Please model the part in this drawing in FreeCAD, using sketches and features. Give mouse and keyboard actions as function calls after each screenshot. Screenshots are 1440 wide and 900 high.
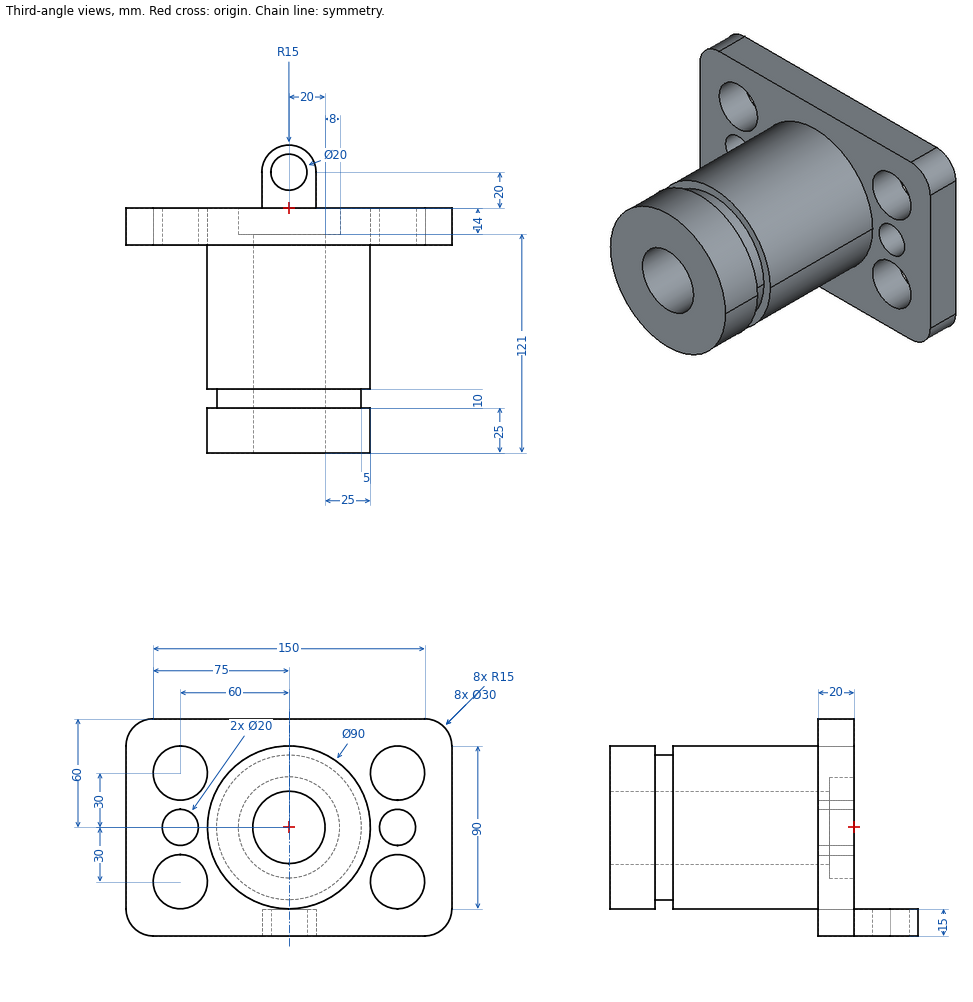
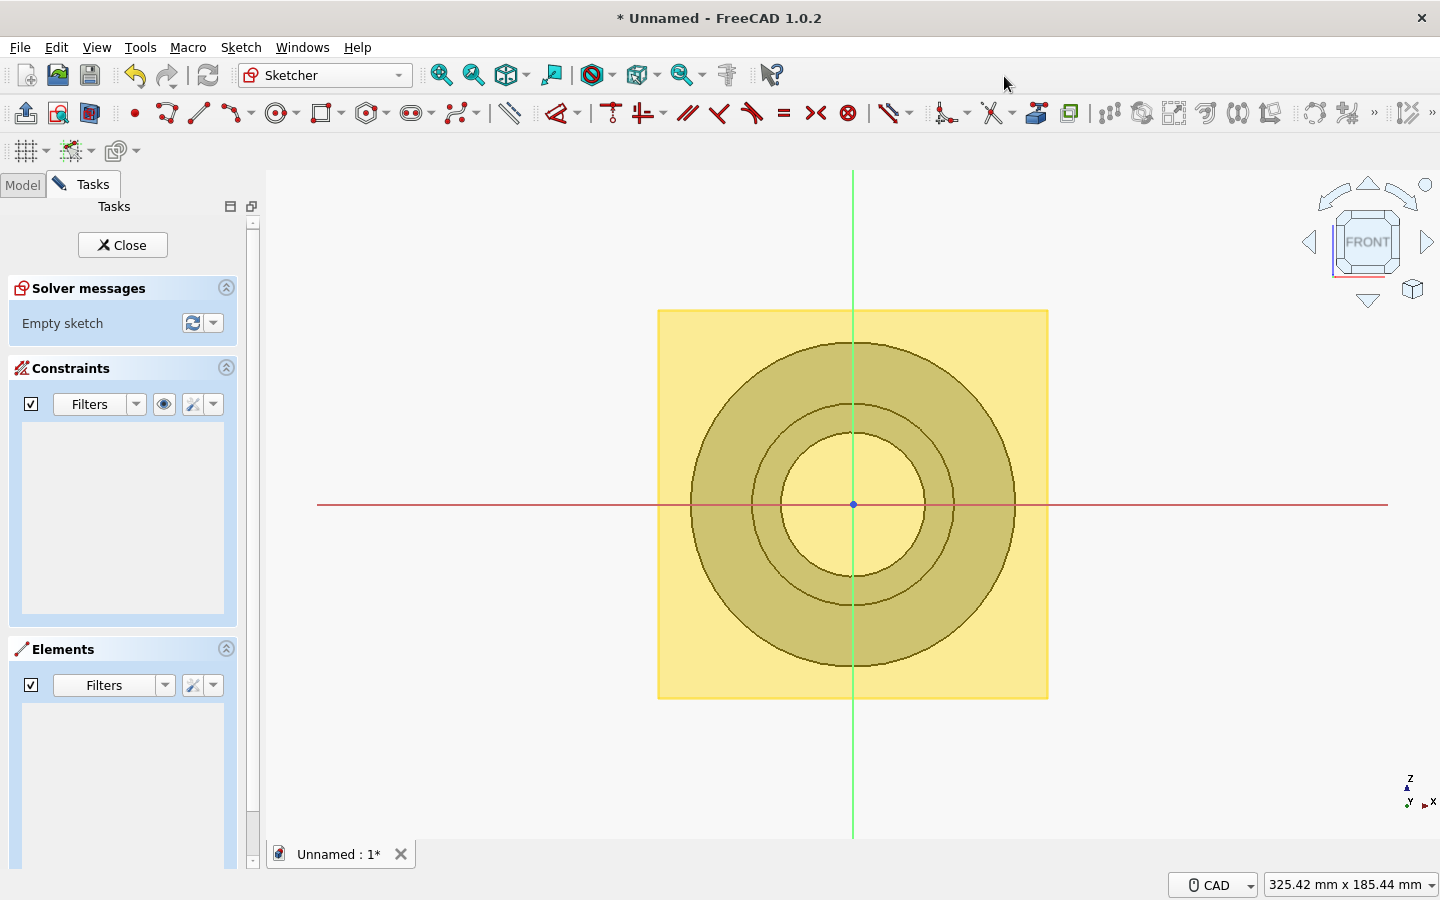
click(200, 114)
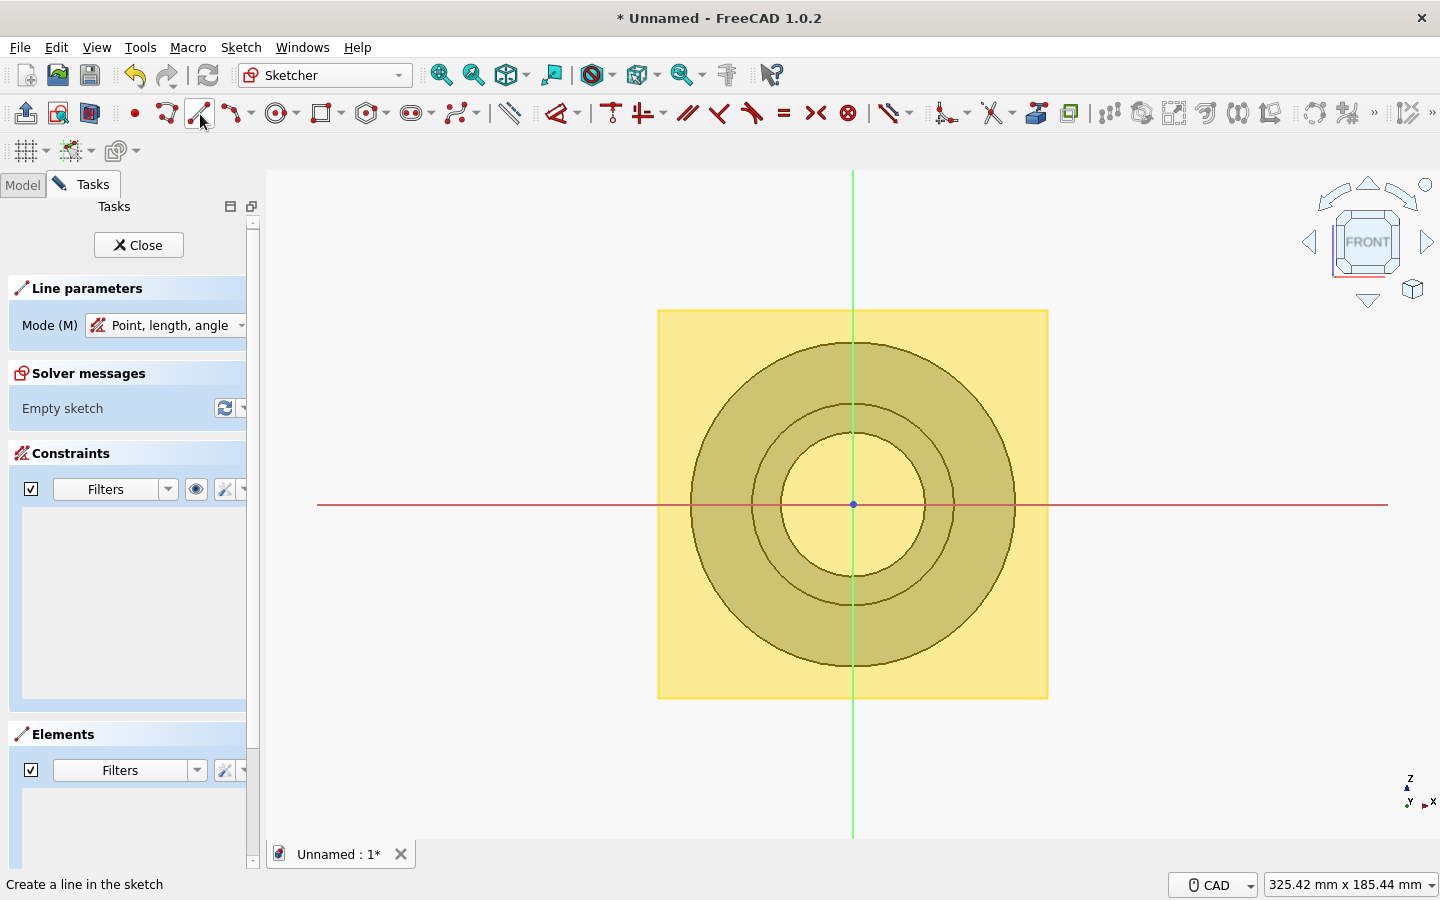
click(582, 288)
click(1124, 288)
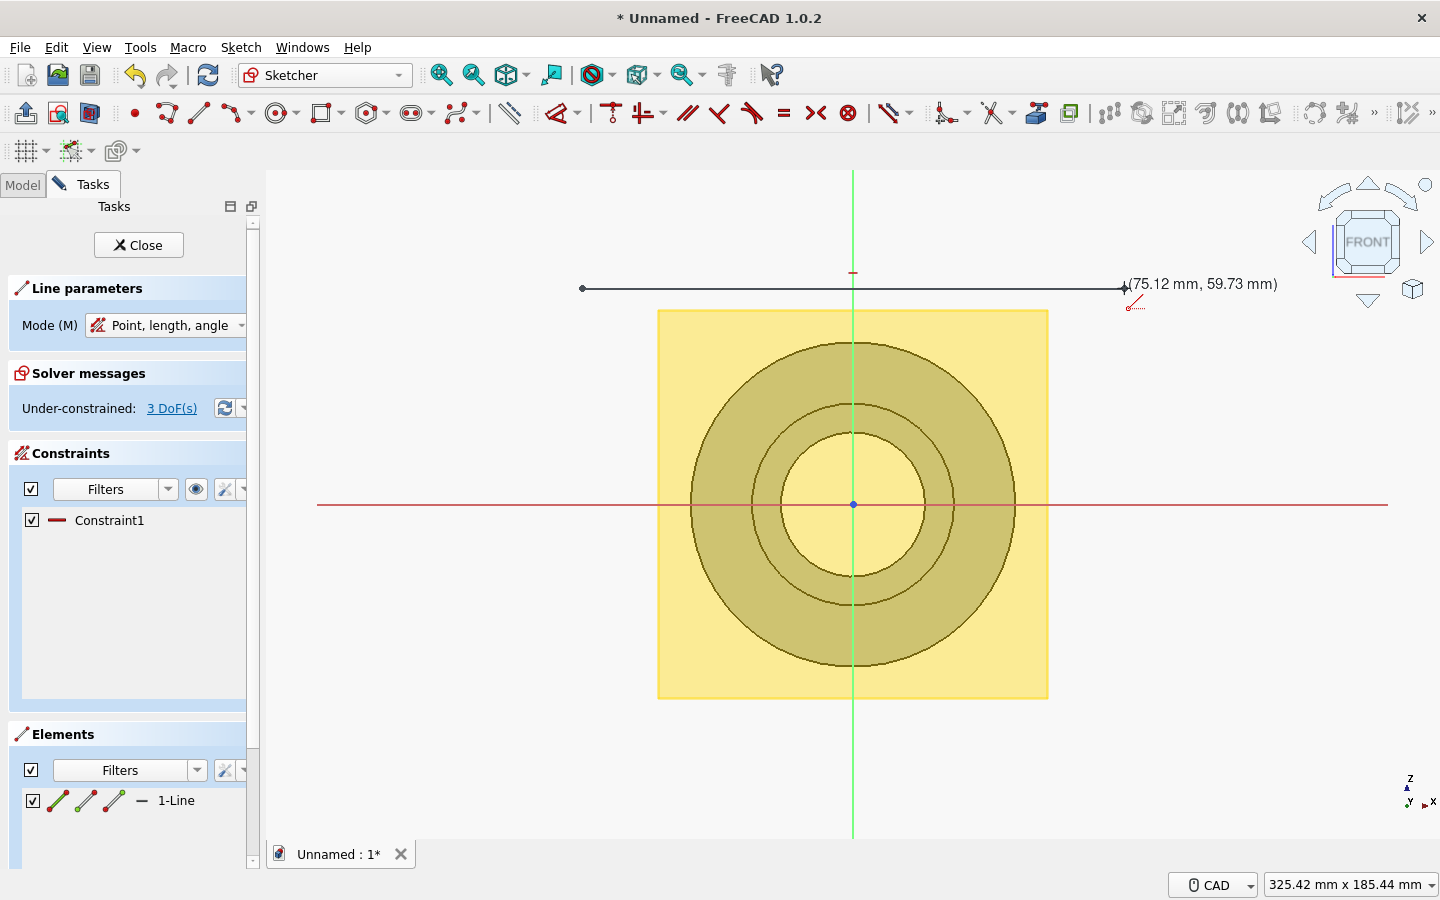
click(1178, 342)
click(1178, 667)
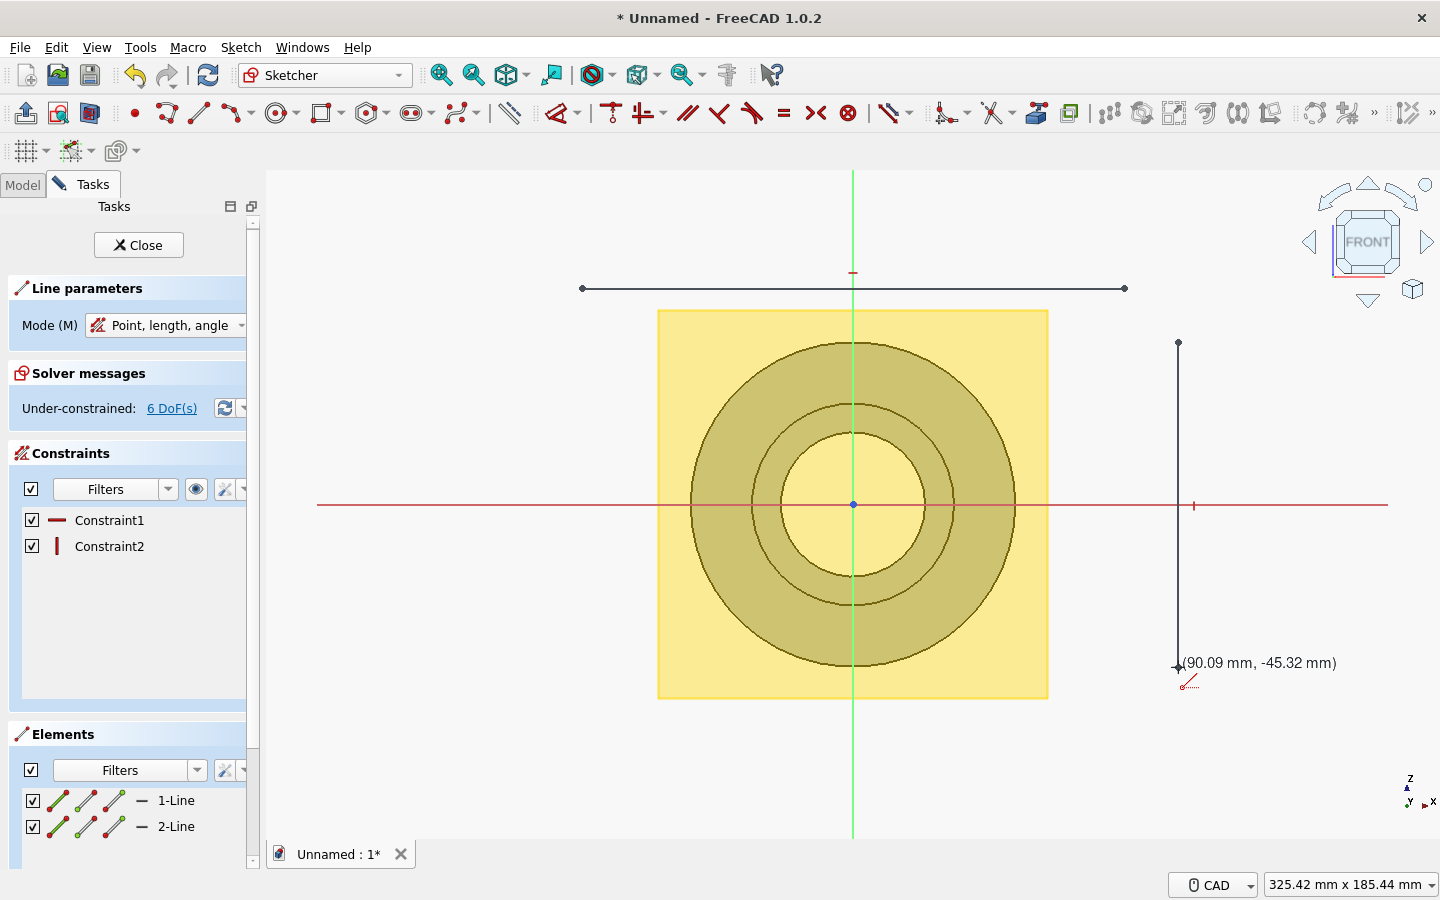
click(1124, 721)
click(582, 721)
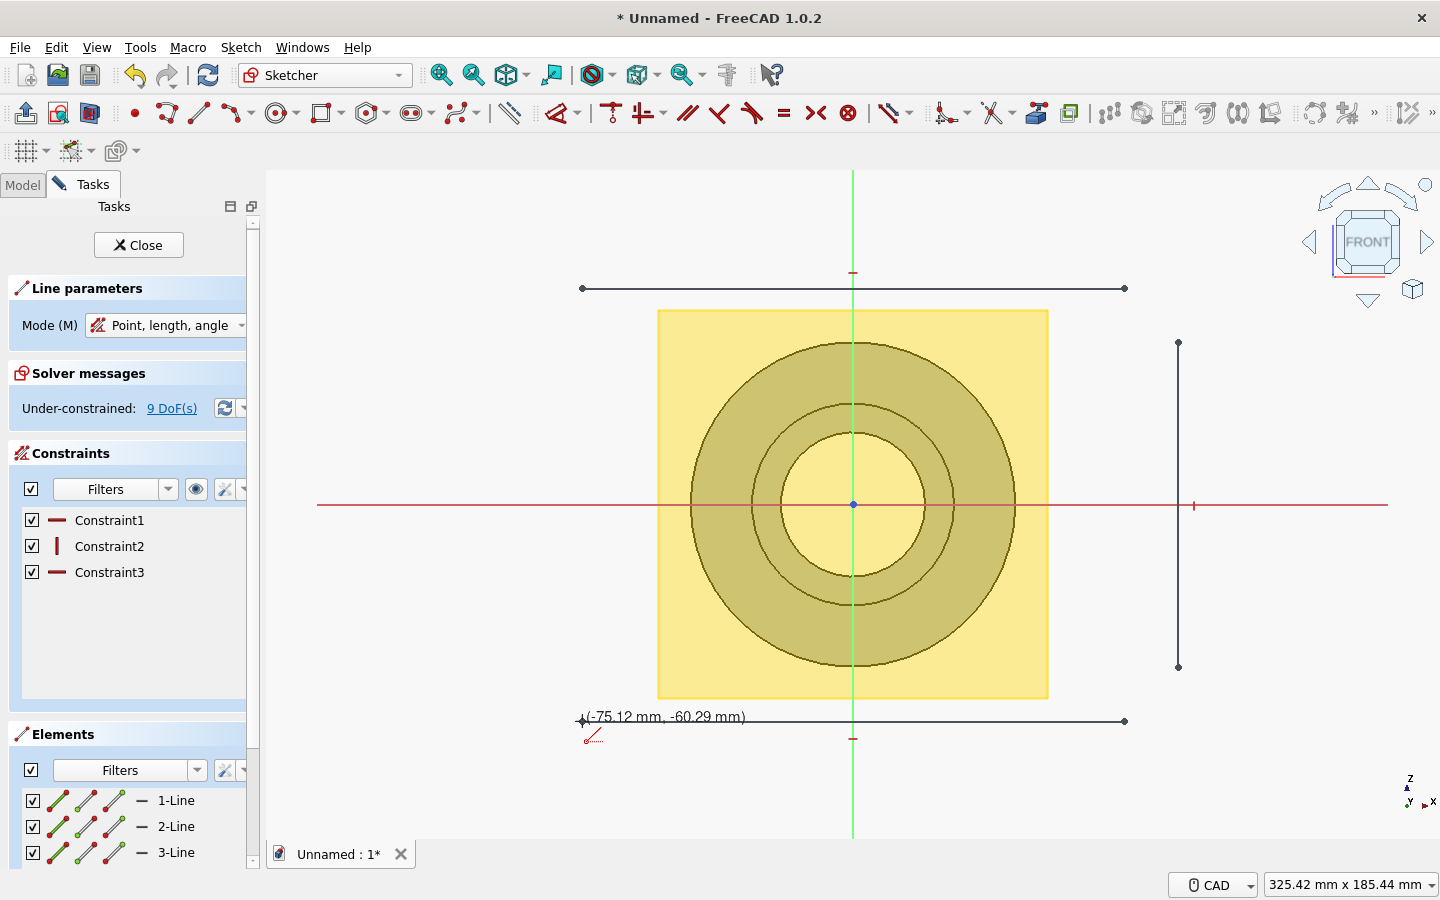
click(528, 667)
click(528, 342)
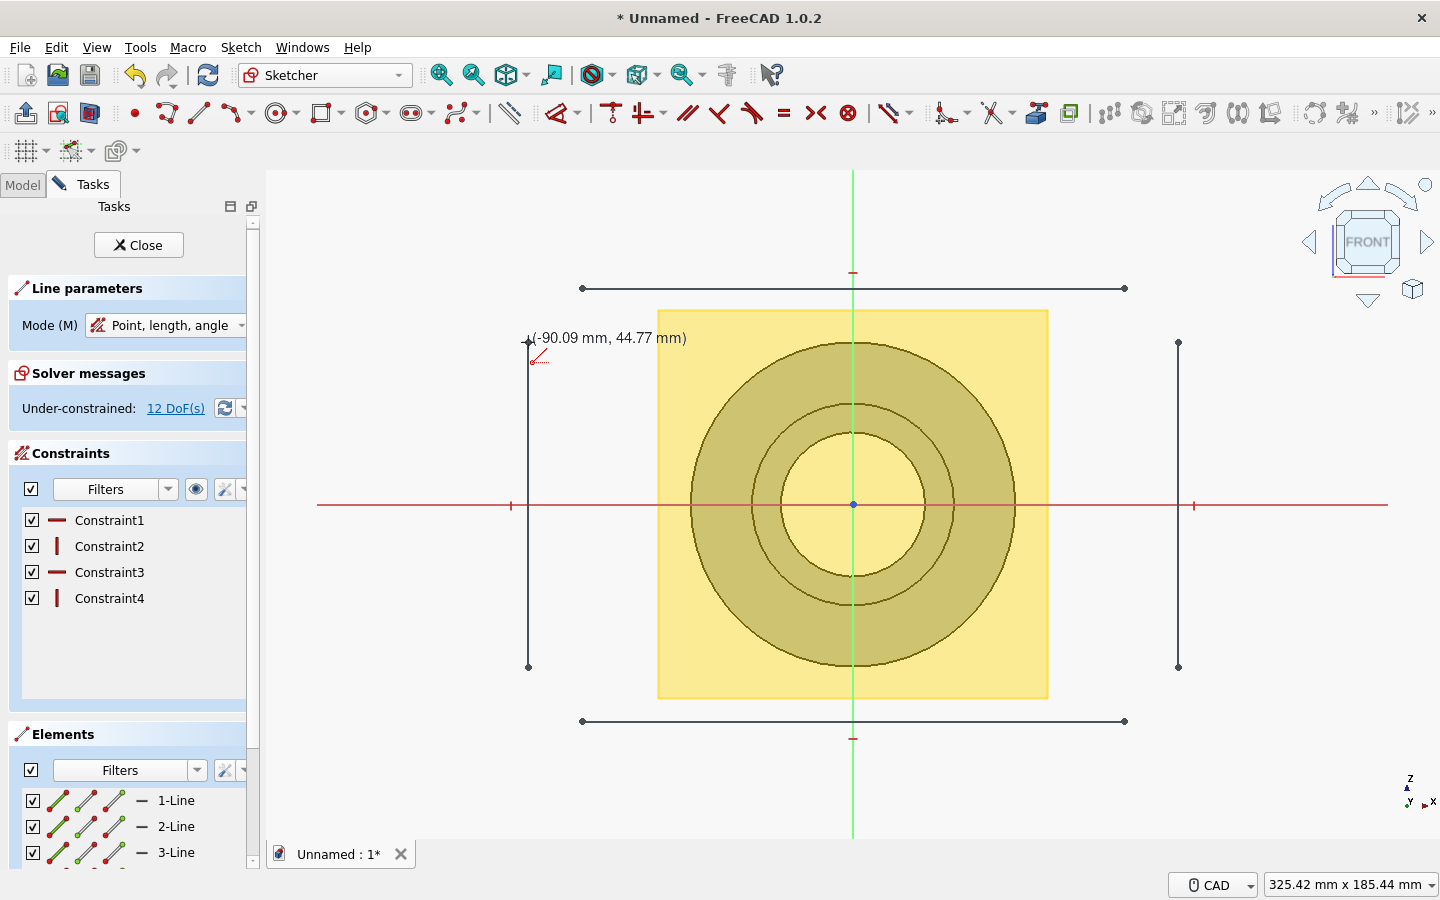
click(232, 114)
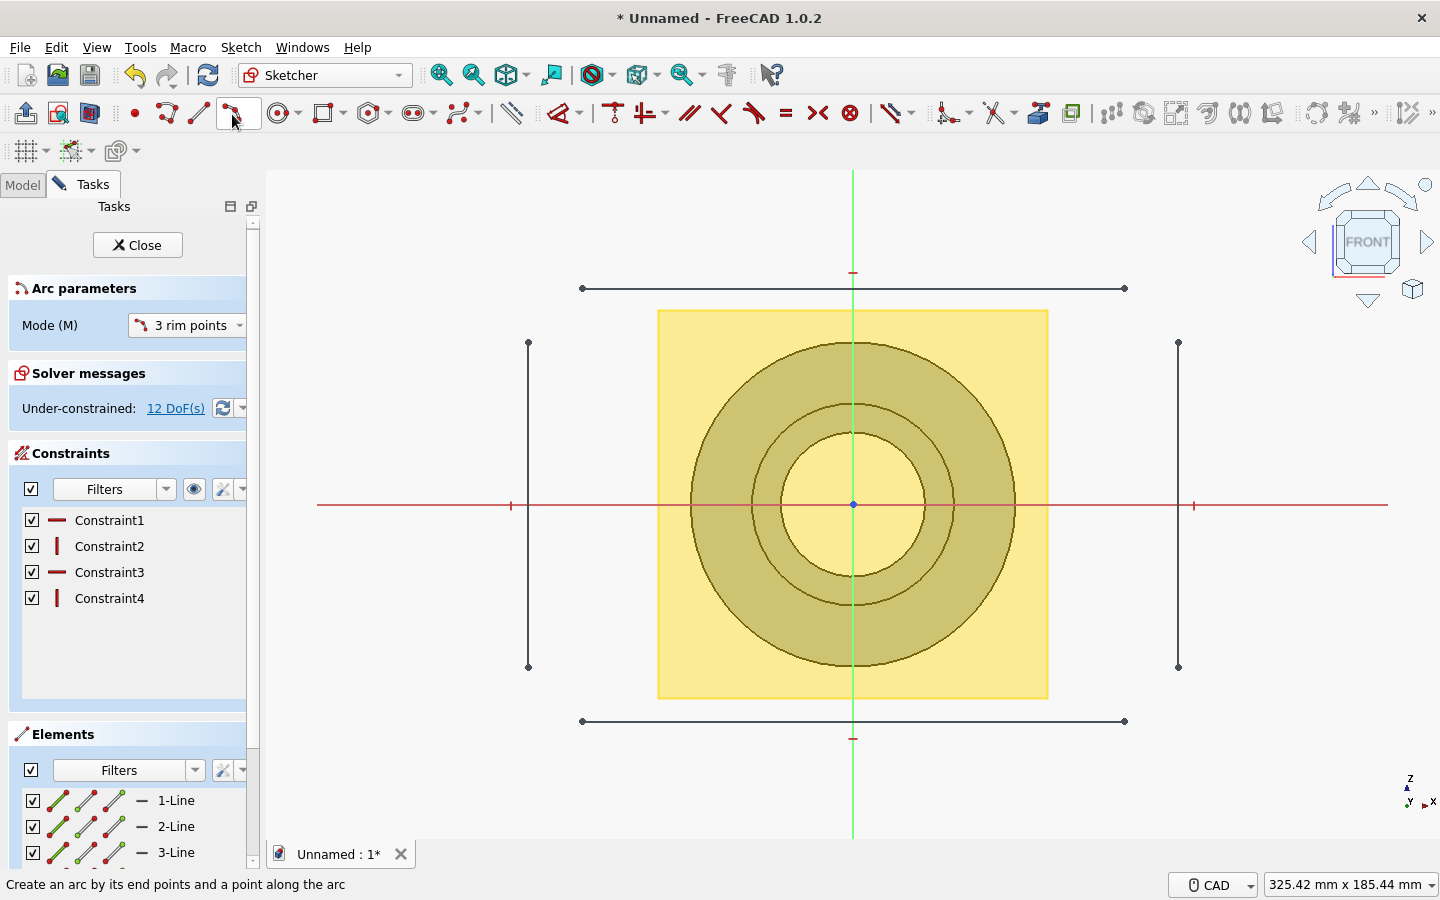
click(1124, 289)
click(1178, 343)
click(1162, 304)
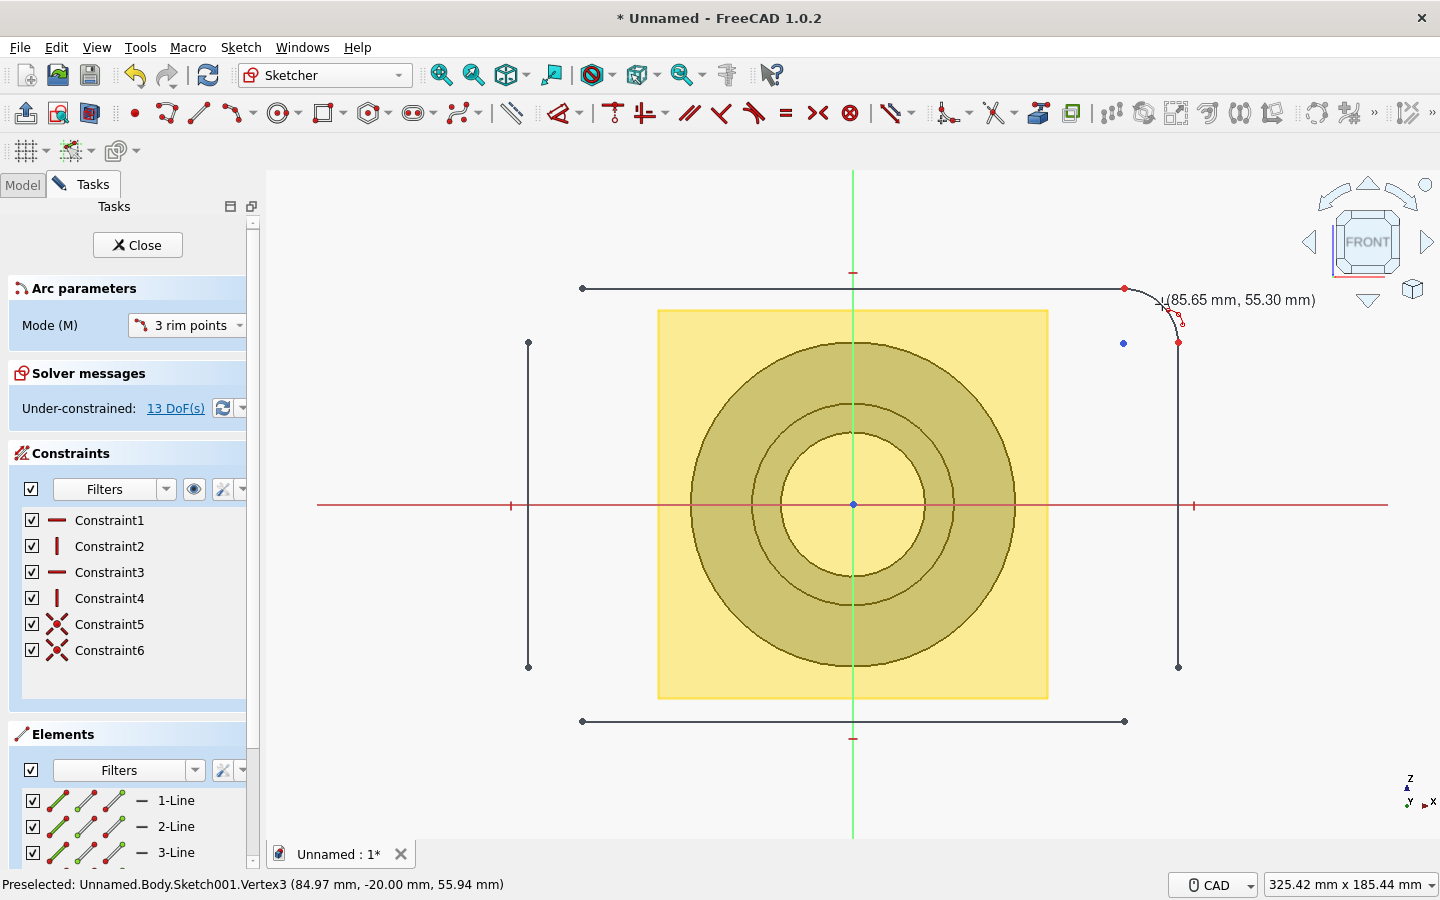
click(1178, 668)
click(1124, 722)
click(1162, 705)